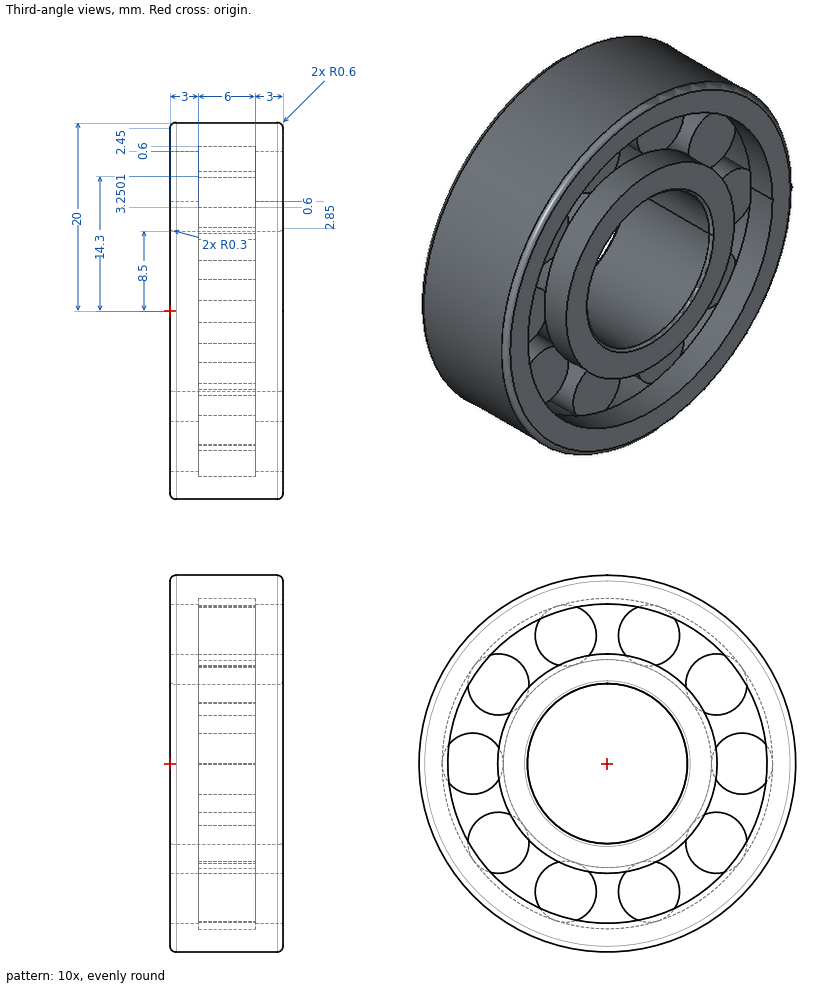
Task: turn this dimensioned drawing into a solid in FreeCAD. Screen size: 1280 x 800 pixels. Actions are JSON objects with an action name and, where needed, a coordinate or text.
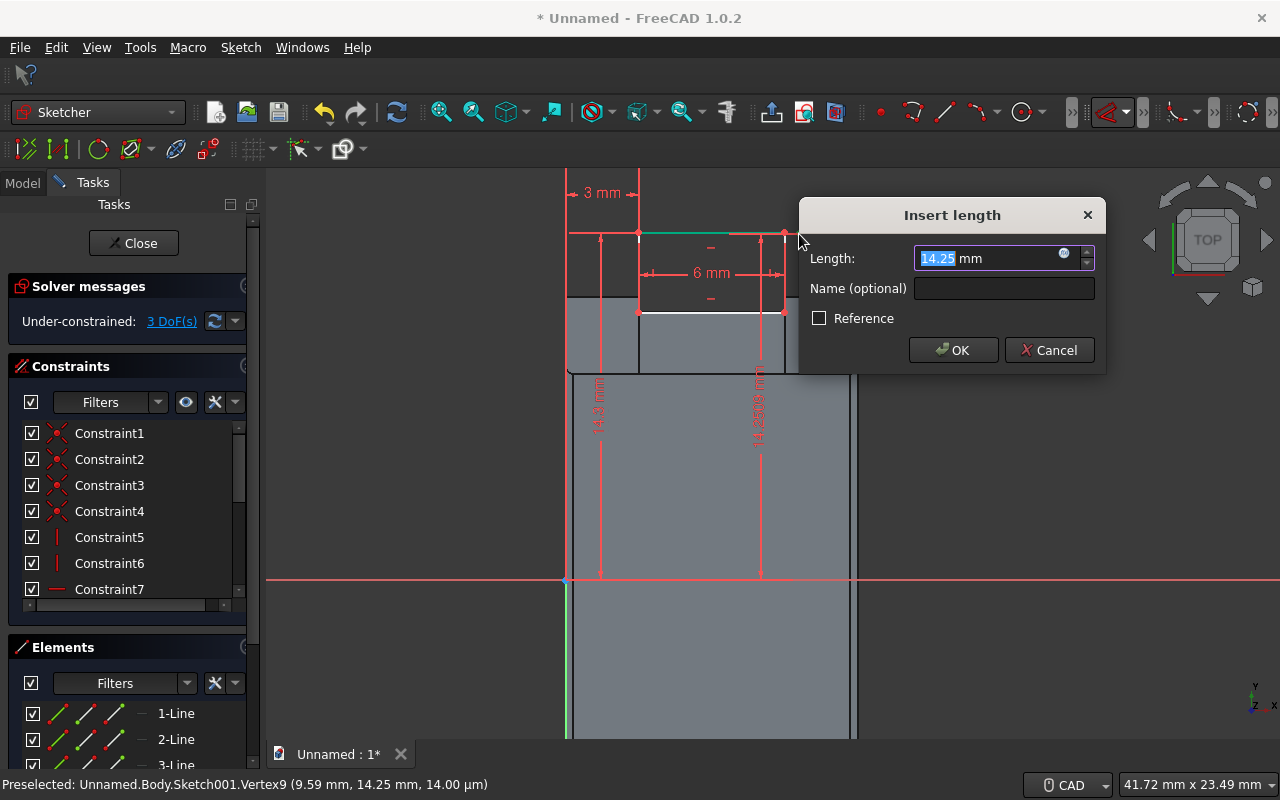
{"action": "type", "text": "14.3"}
{"action": "key", "text": "Return"}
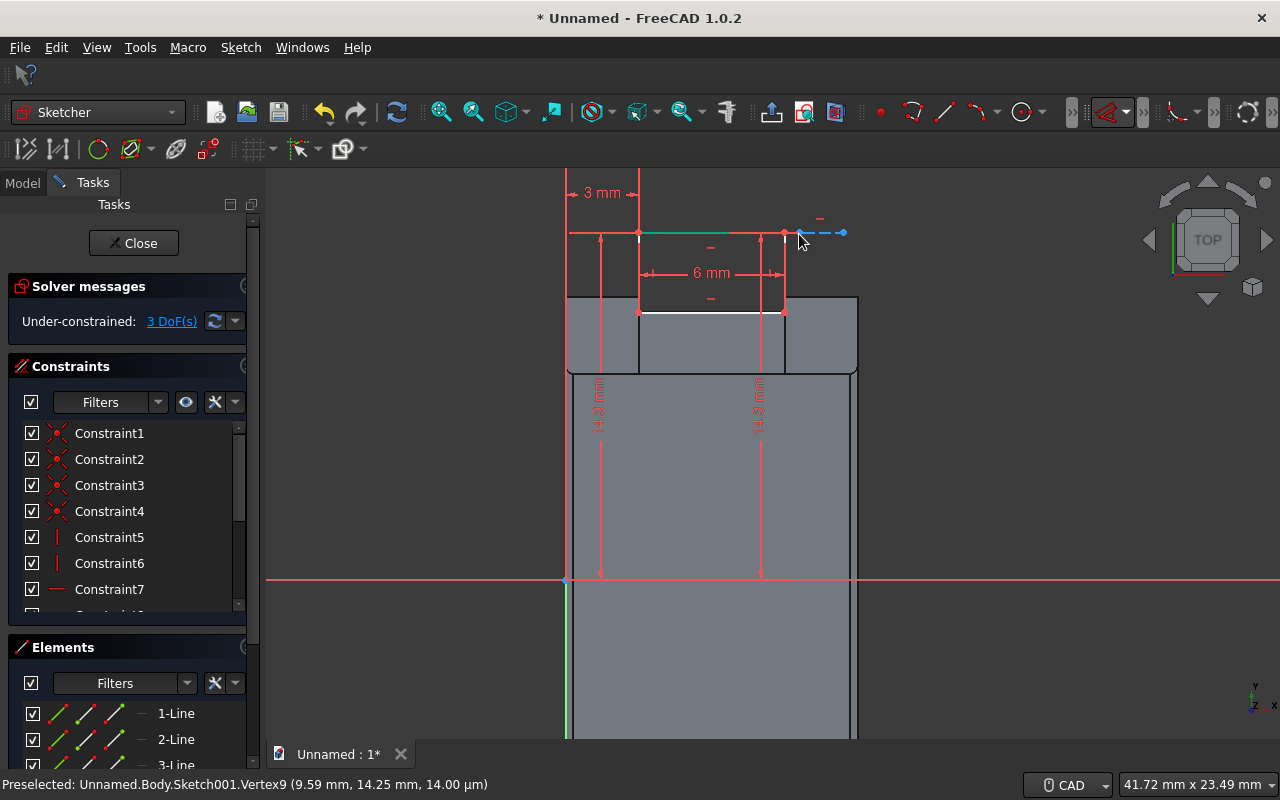
{"action": "left_click", "coordinate": [639, 257]}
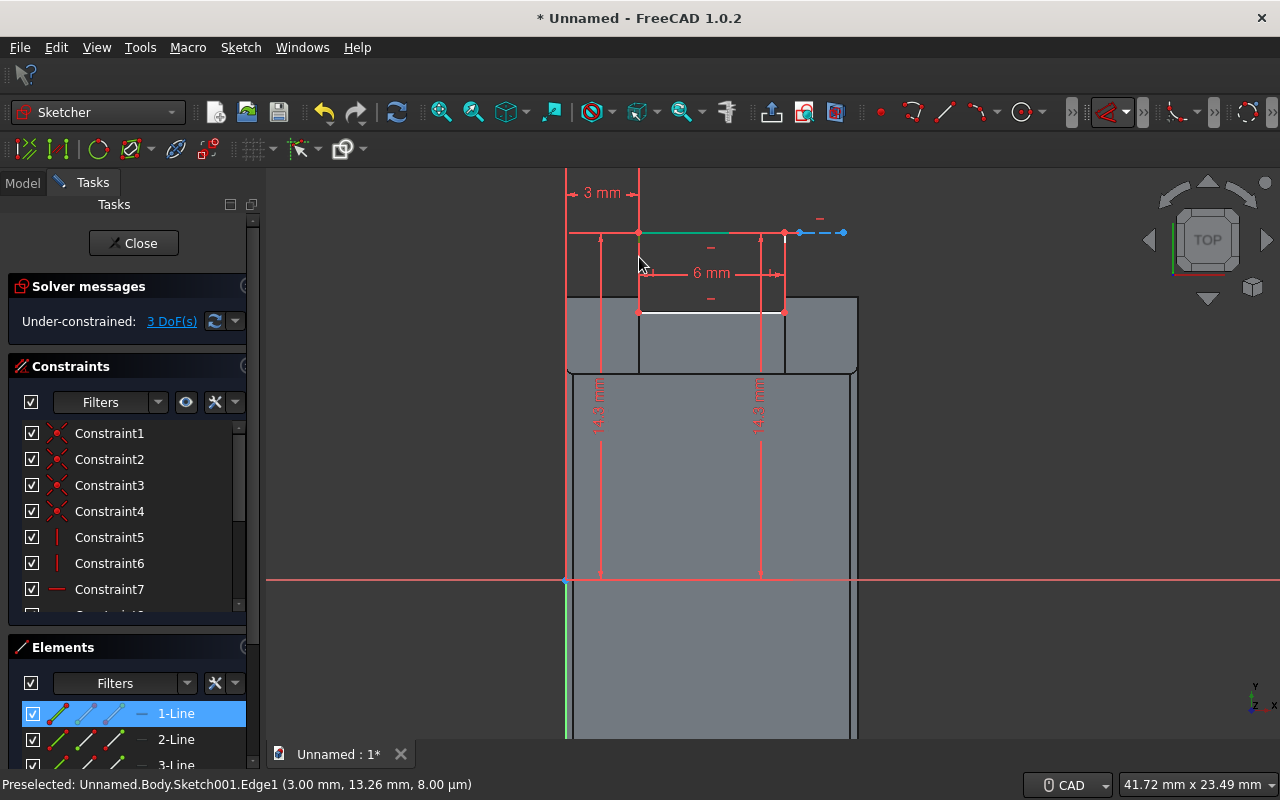
{"action": "key", "text": "i"}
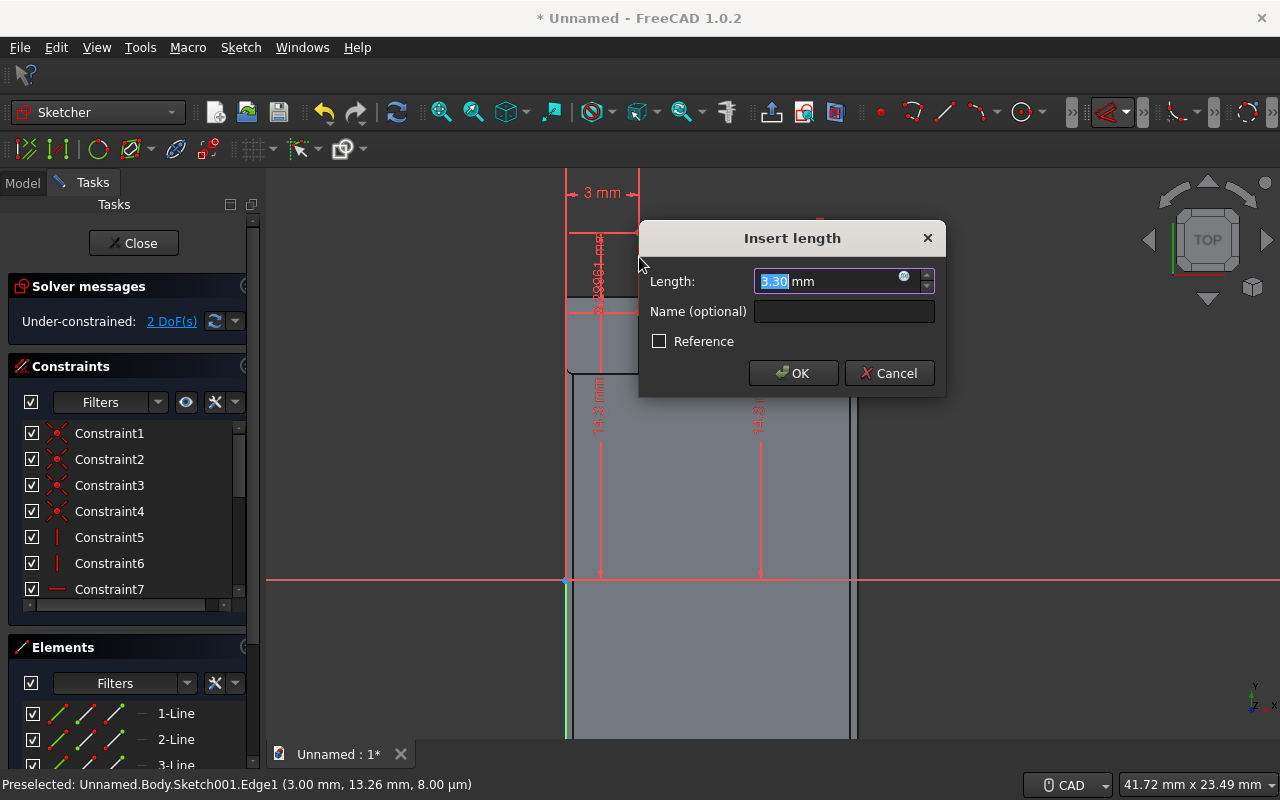
{"action": "type", "text": "3.2501"}
{"action": "key", "text": "Return"}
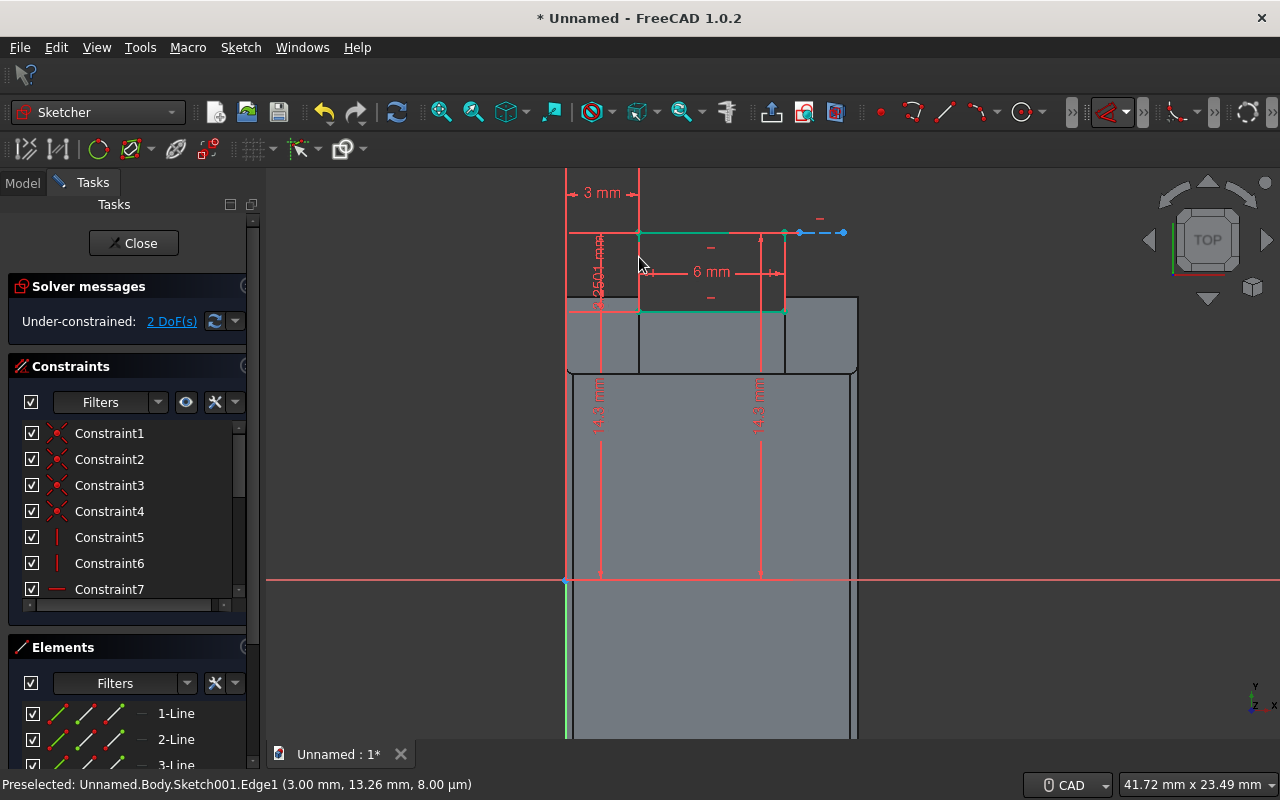
{"action": "left_click", "coordinate": [134, 243]}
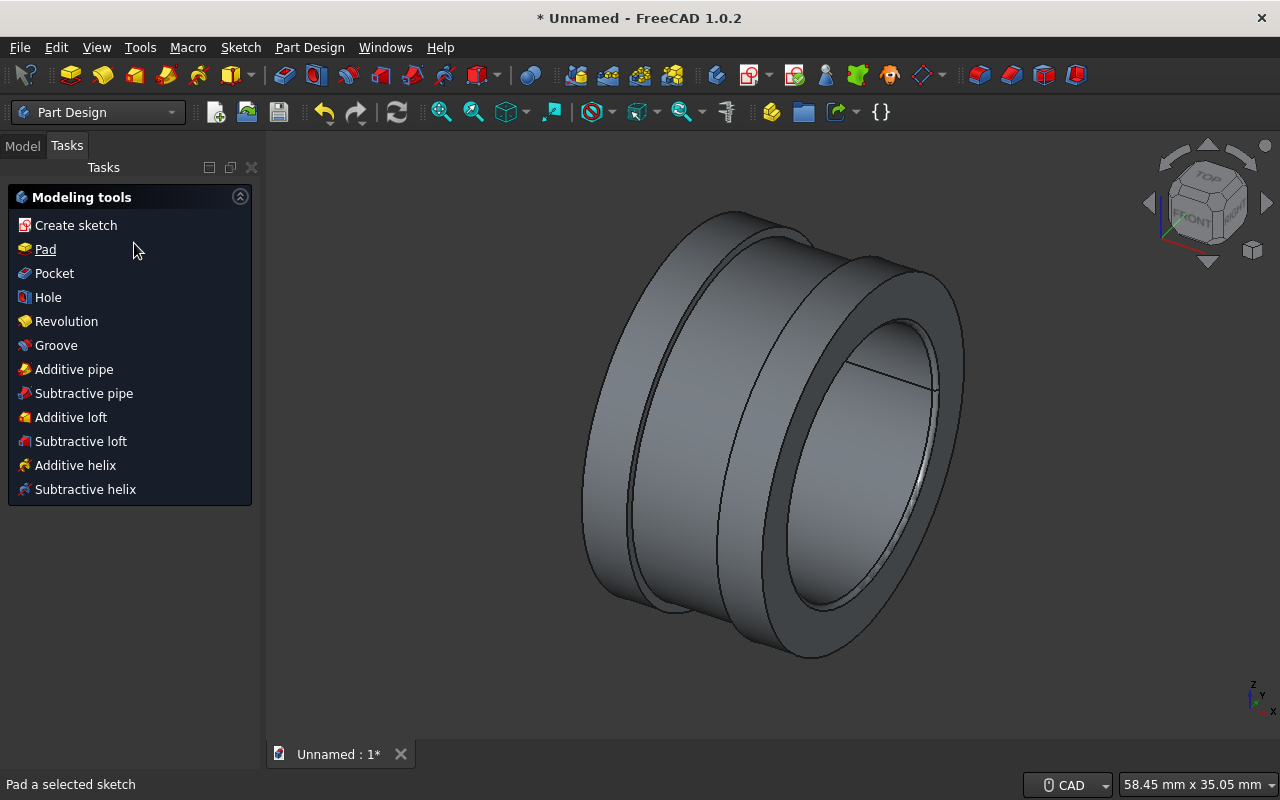
{"action": "left_click", "coordinate": [104, 76]}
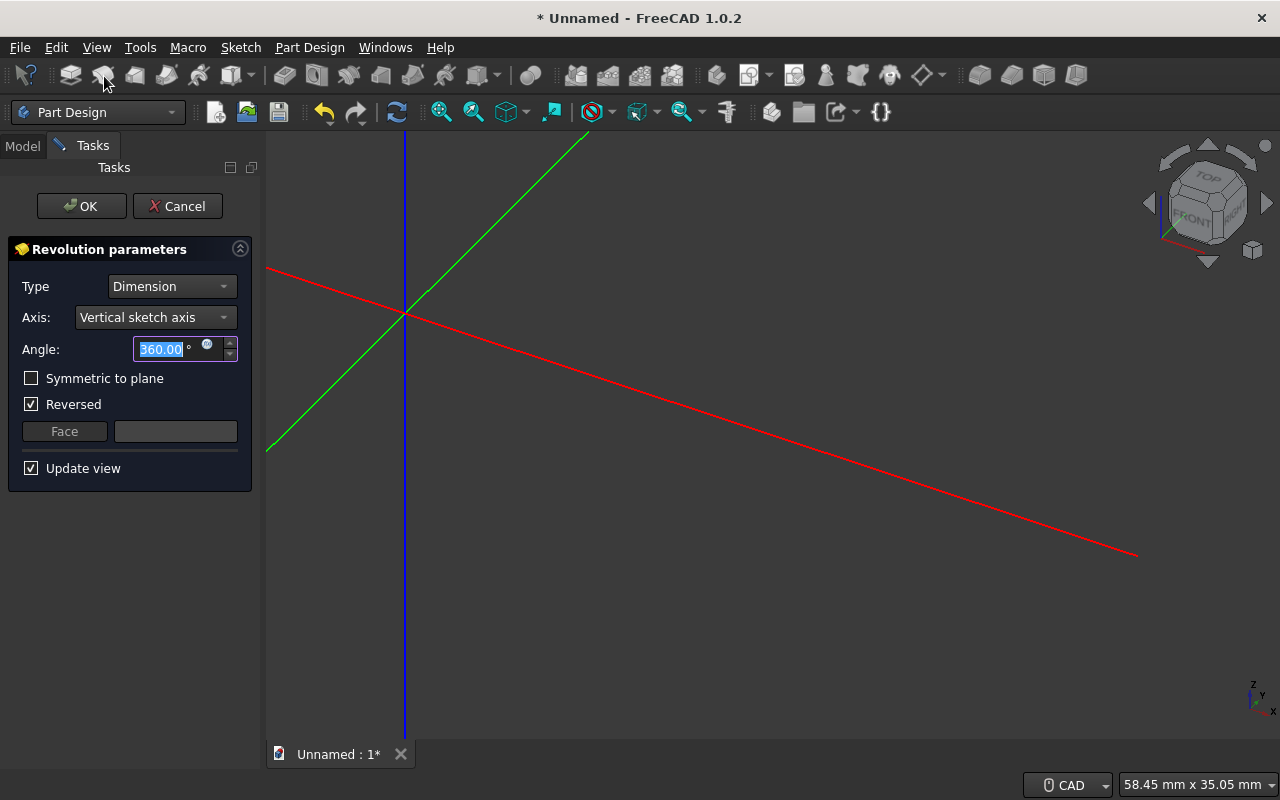
{"action": "left_click", "coordinate": [156, 318]}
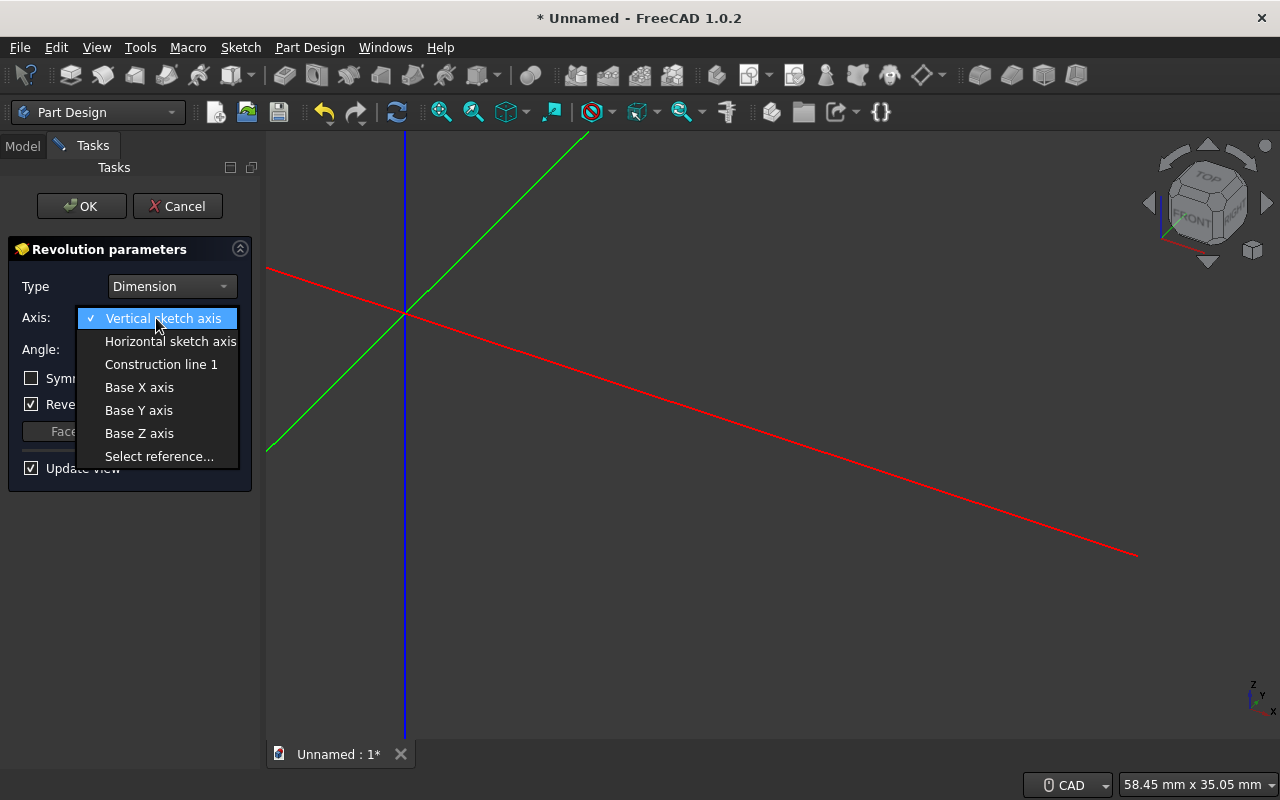
{"action": "left_click", "coordinate": [156, 364]}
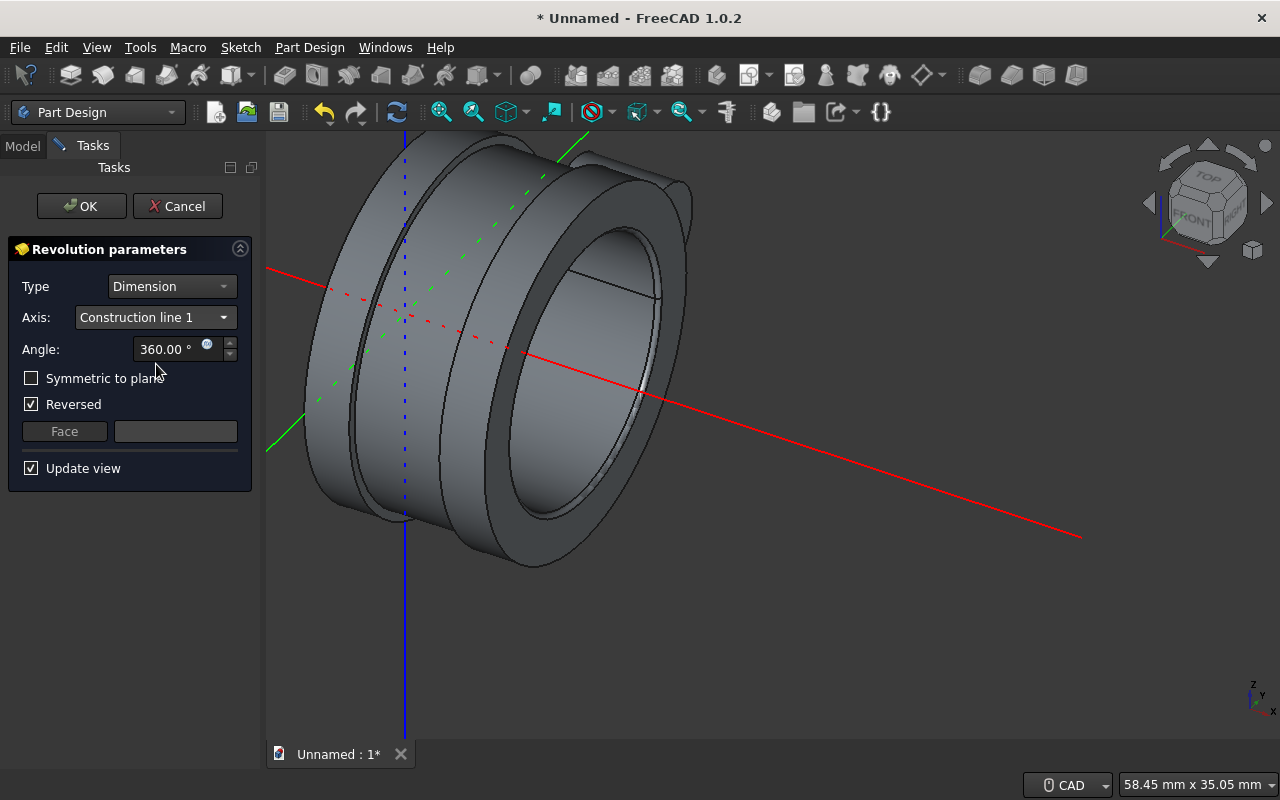
{"action": "left_click", "coordinate": [82, 206]}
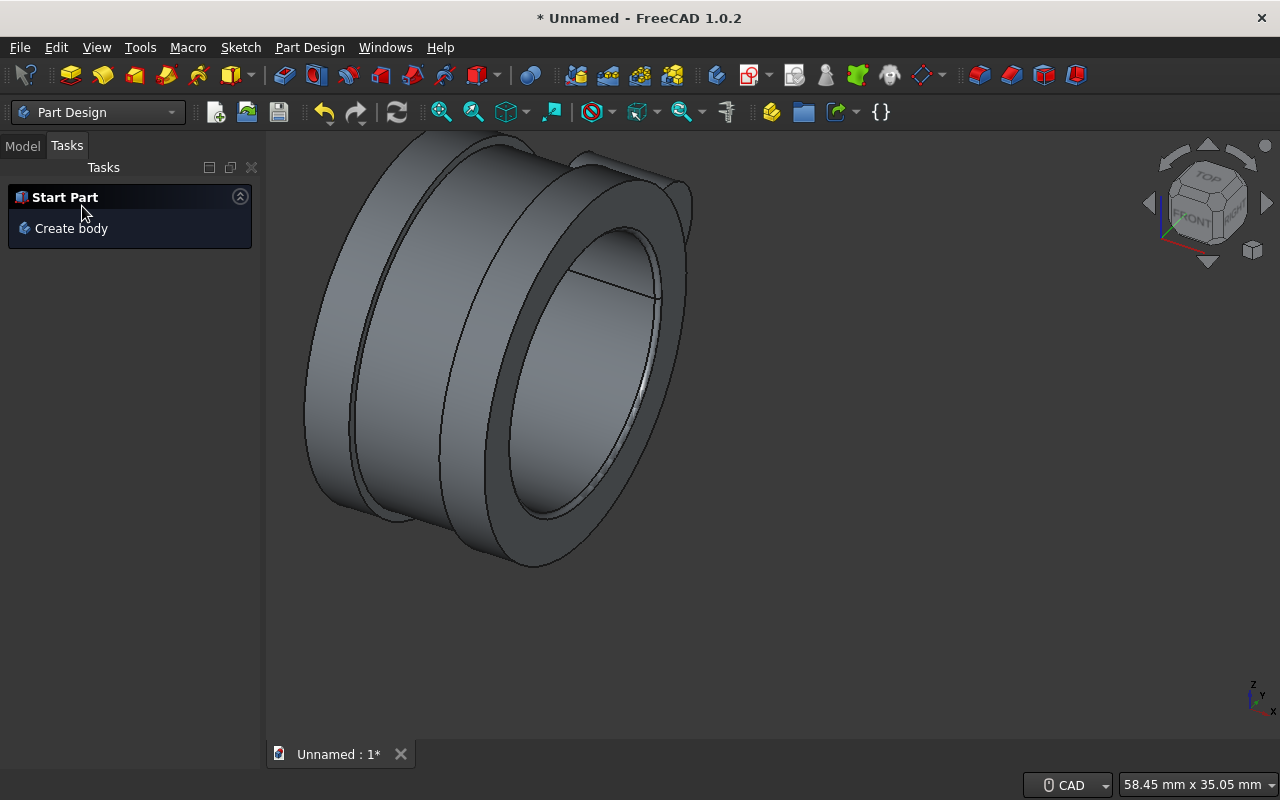
{"action": "key", "text": "v f"}